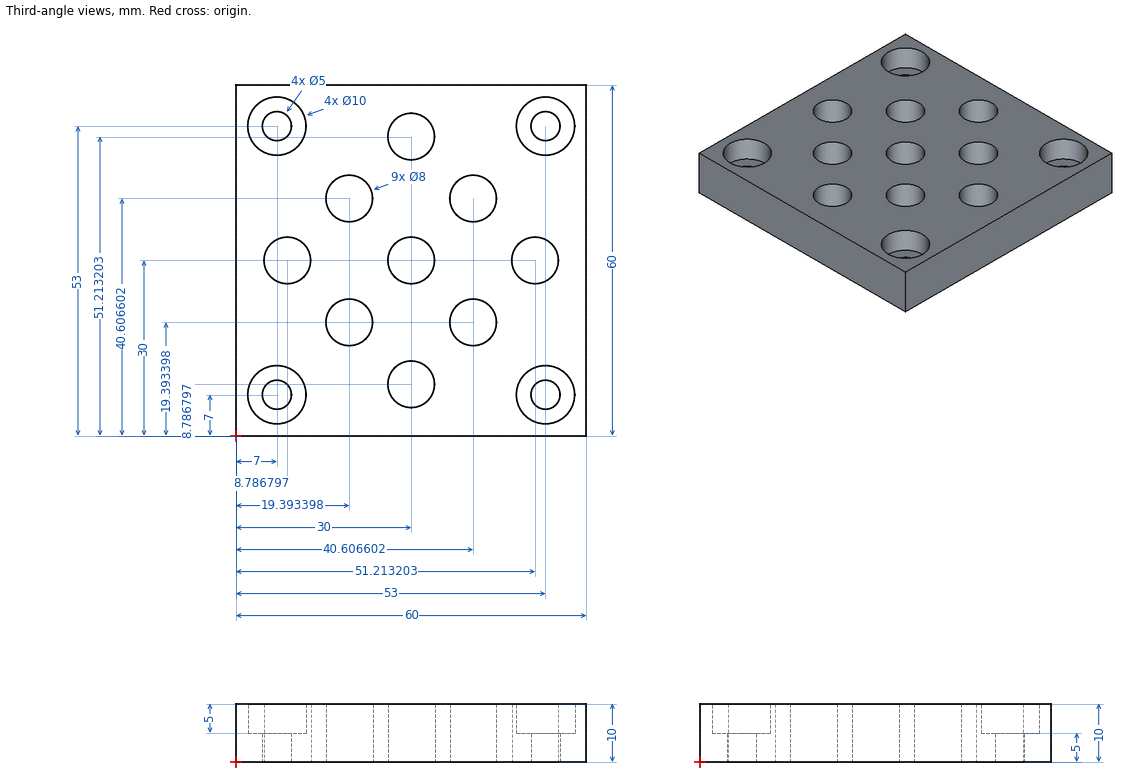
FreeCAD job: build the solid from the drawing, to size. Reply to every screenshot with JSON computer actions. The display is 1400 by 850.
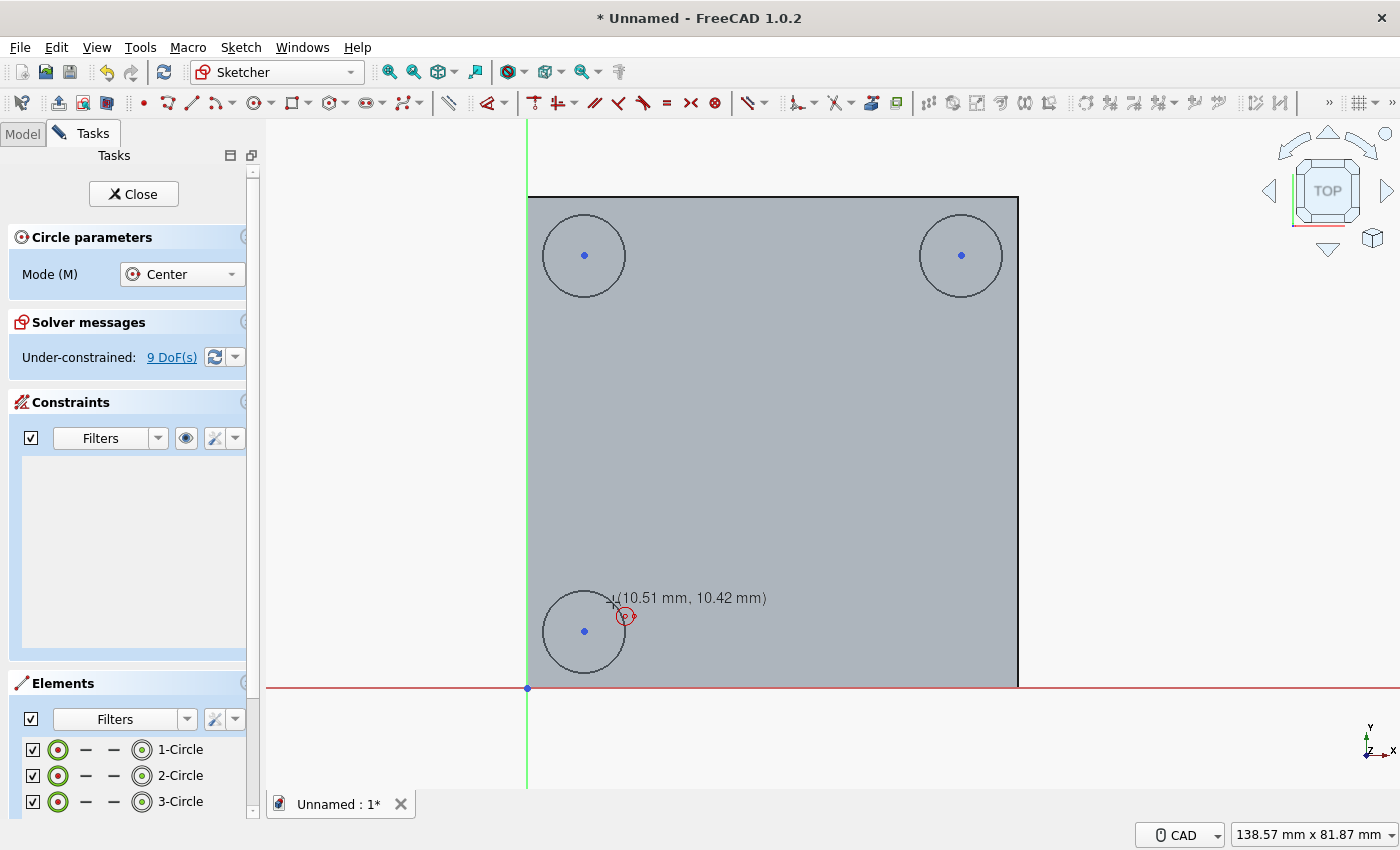
{"action": "left_click", "coordinate": [961, 631]}
{"action": "left_click", "coordinate": [990, 602]}
{"action": "key", "text": "Escape"}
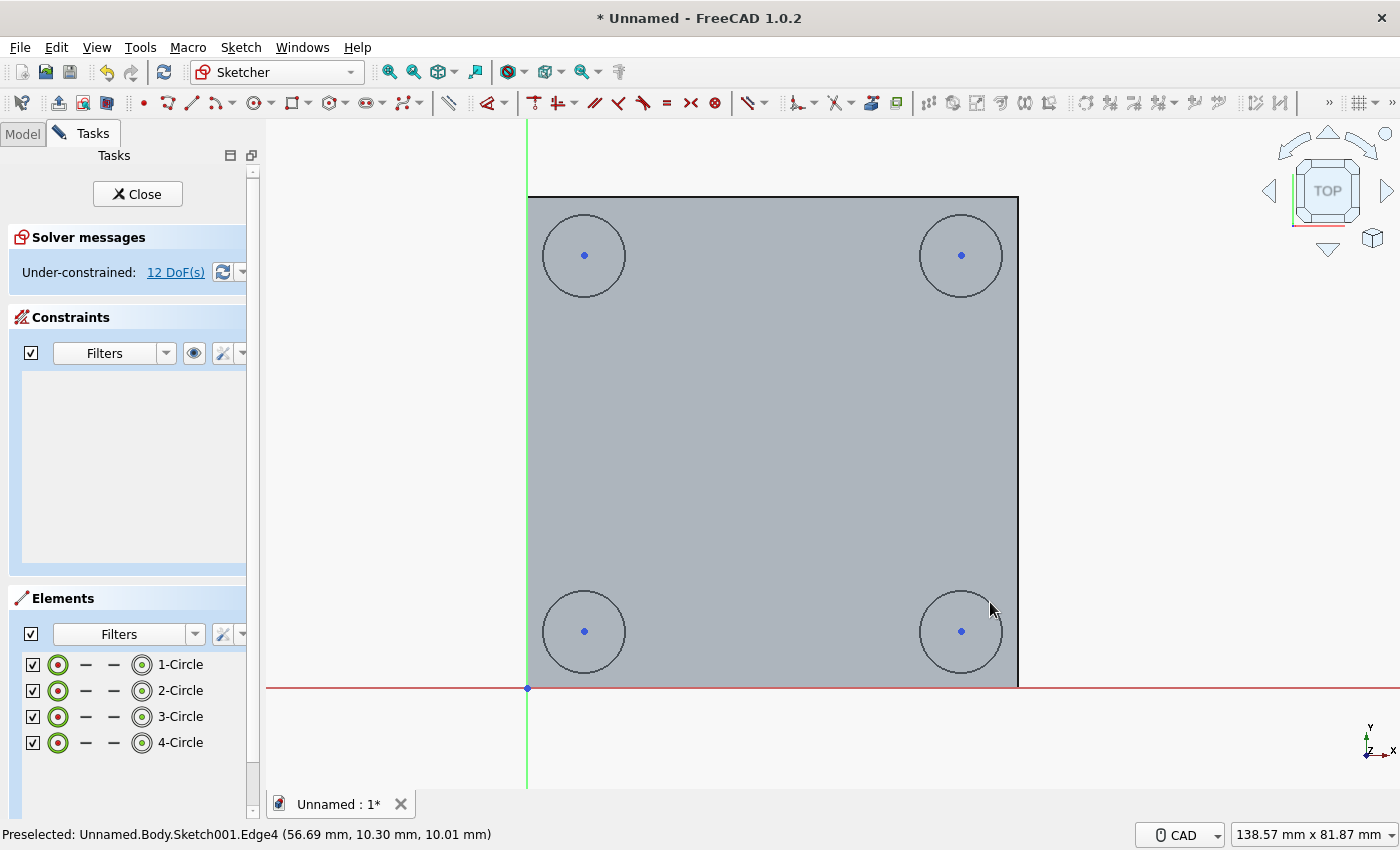
{"action": "left_click", "coordinate": [613, 227]}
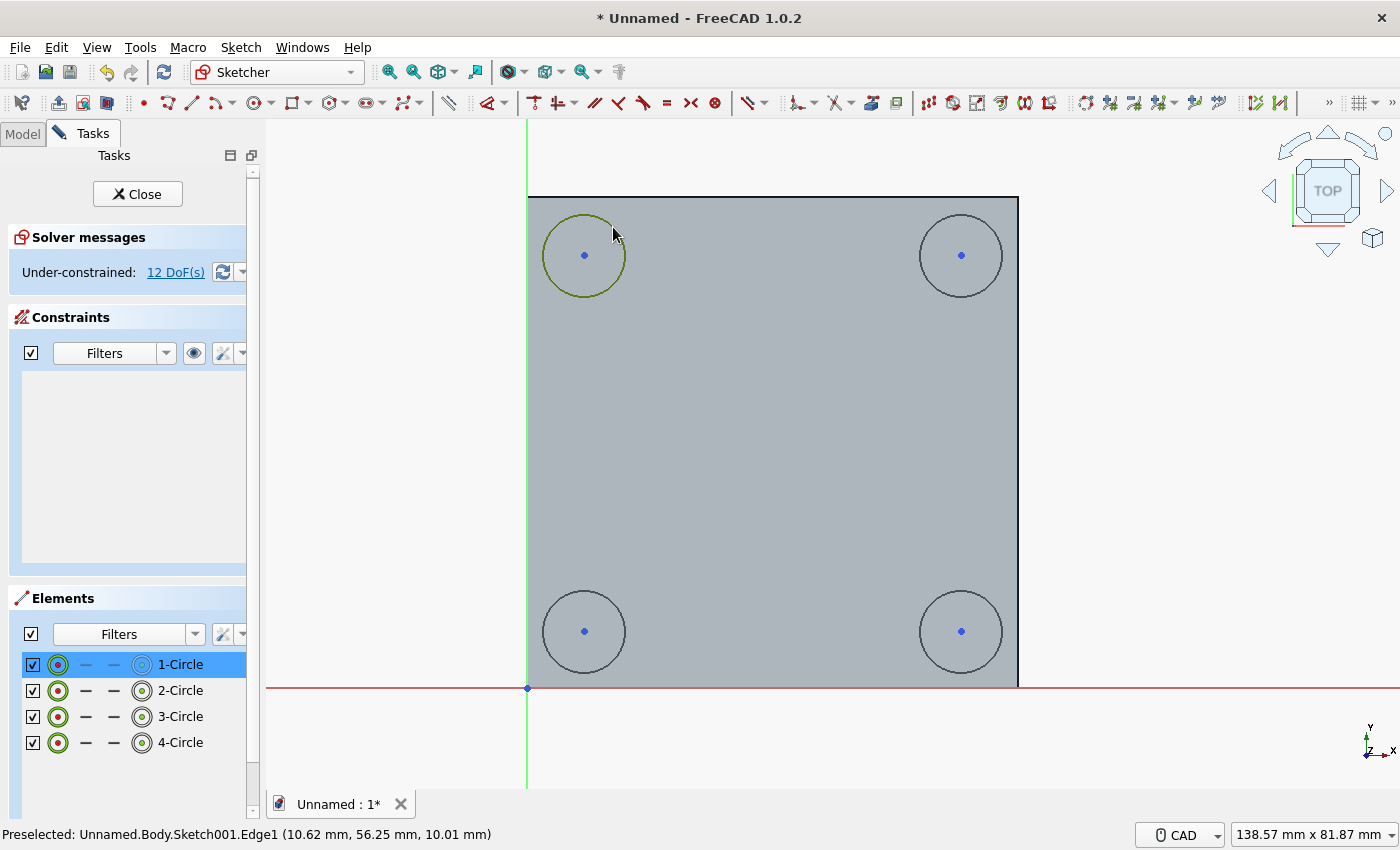
{"action": "left_click", "coordinate": [990, 227]}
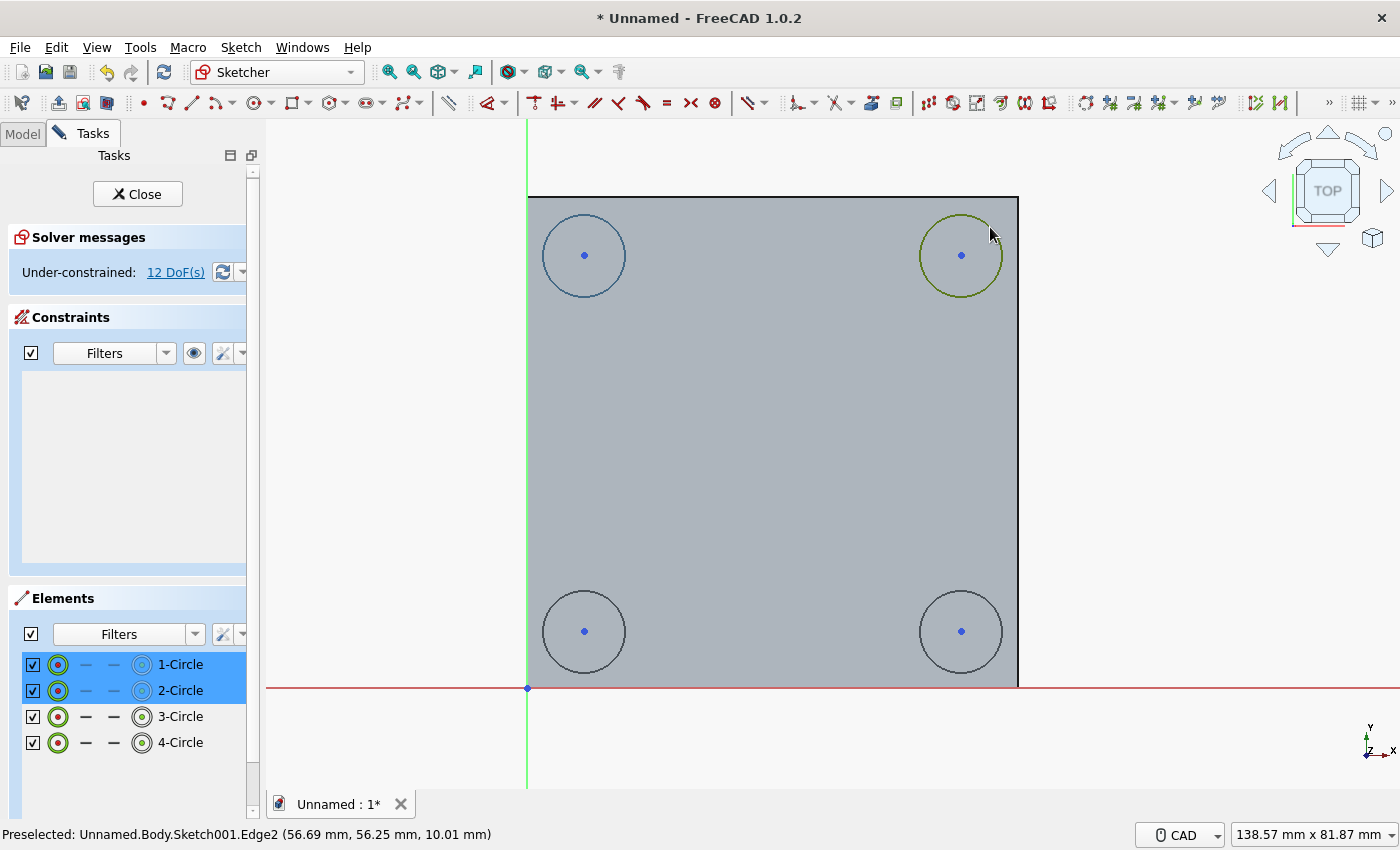
{"action": "left_click", "coordinate": [613, 603]}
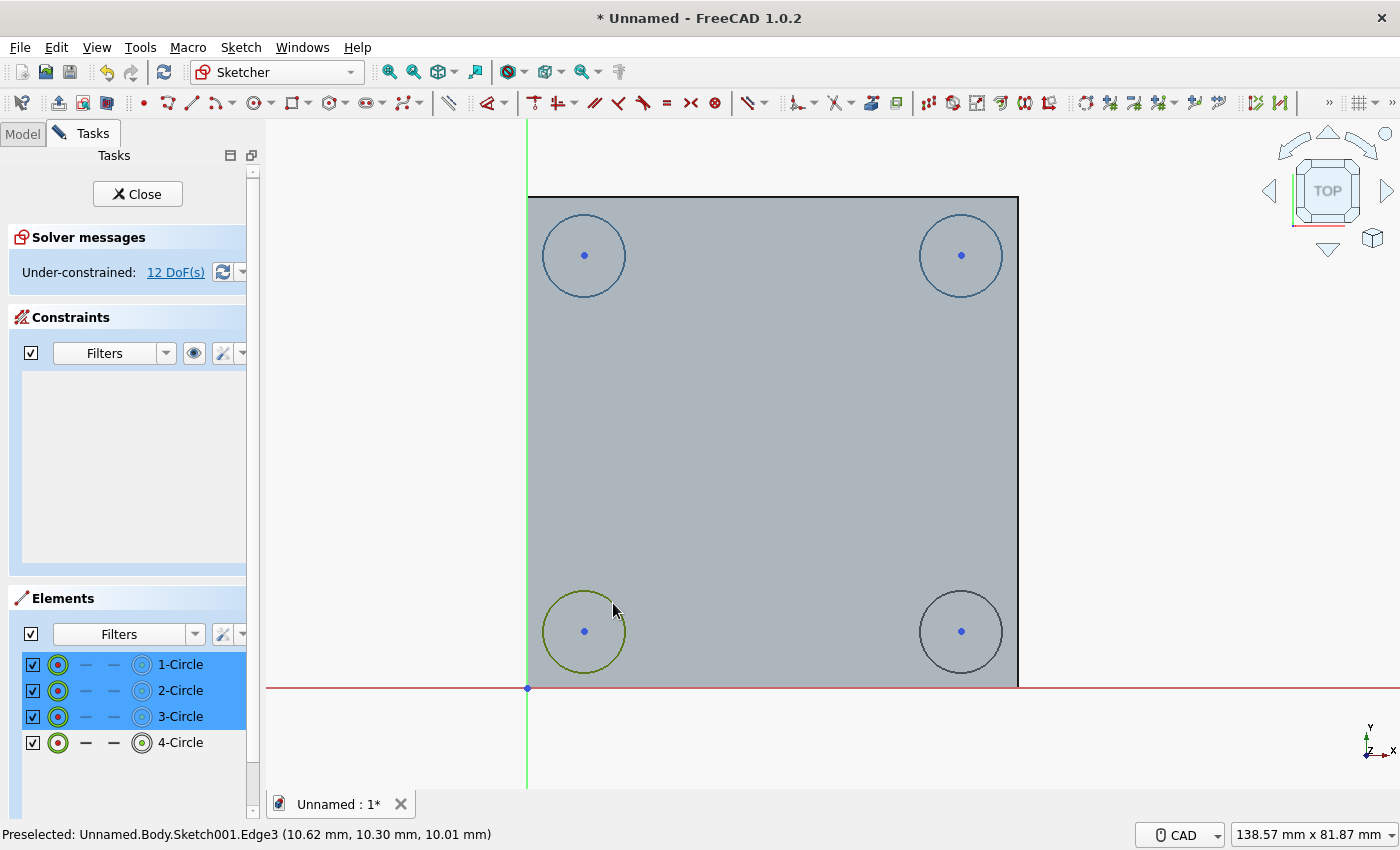
{"action": "left_click", "coordinate": [990, 603]}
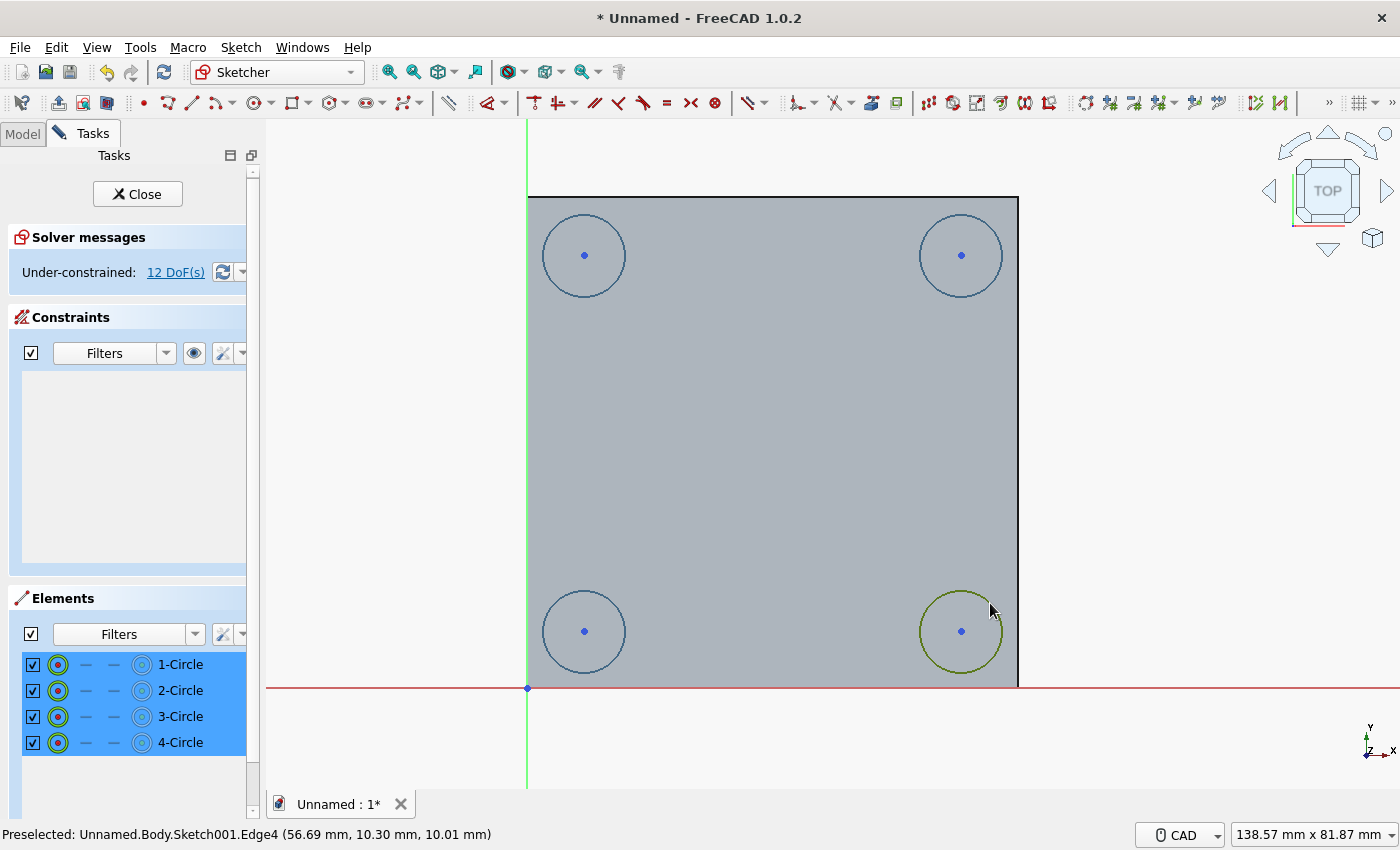
{"action": "key", "text": "e"}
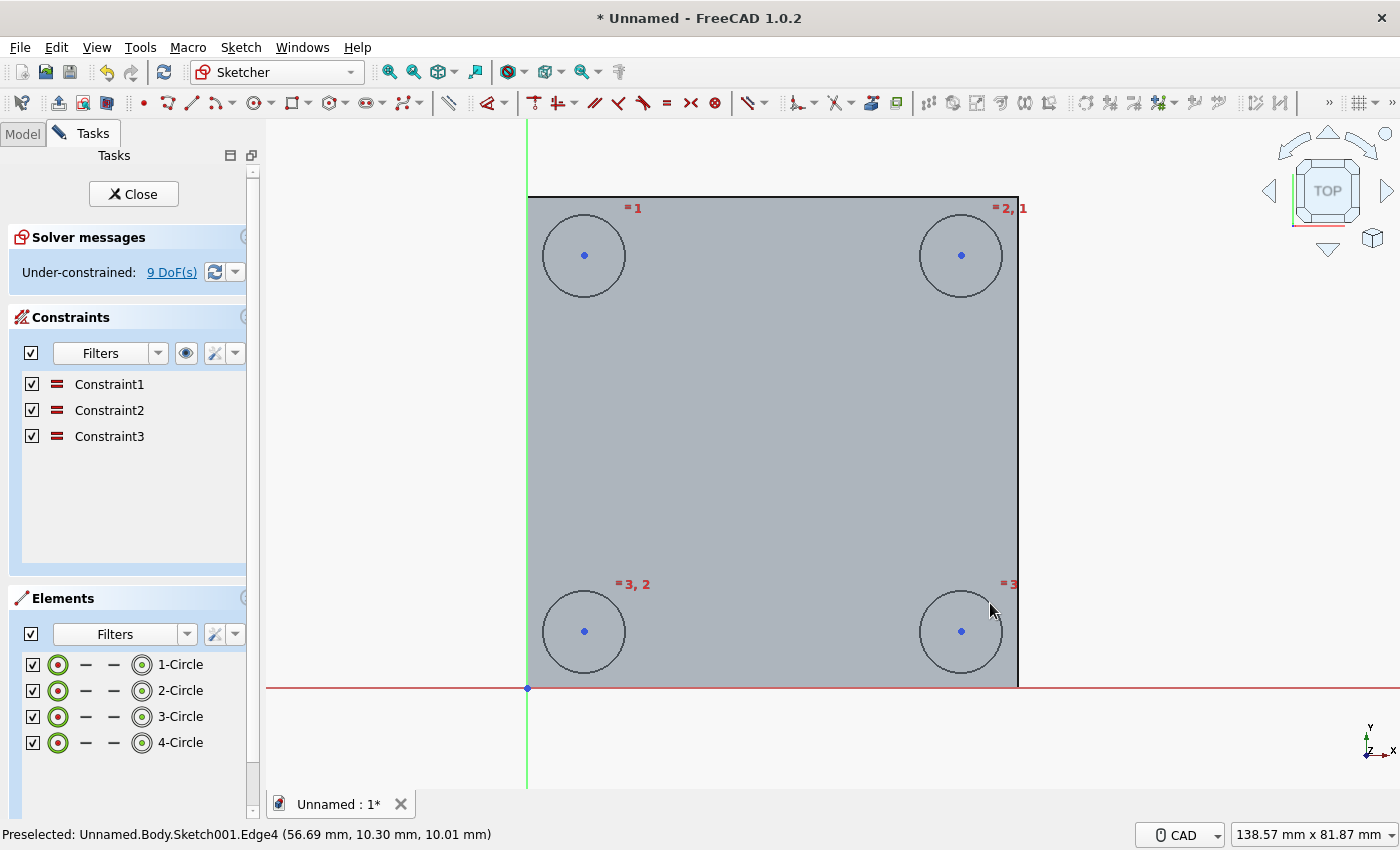
{"action": "left_click", "coordinate": [584, 256]}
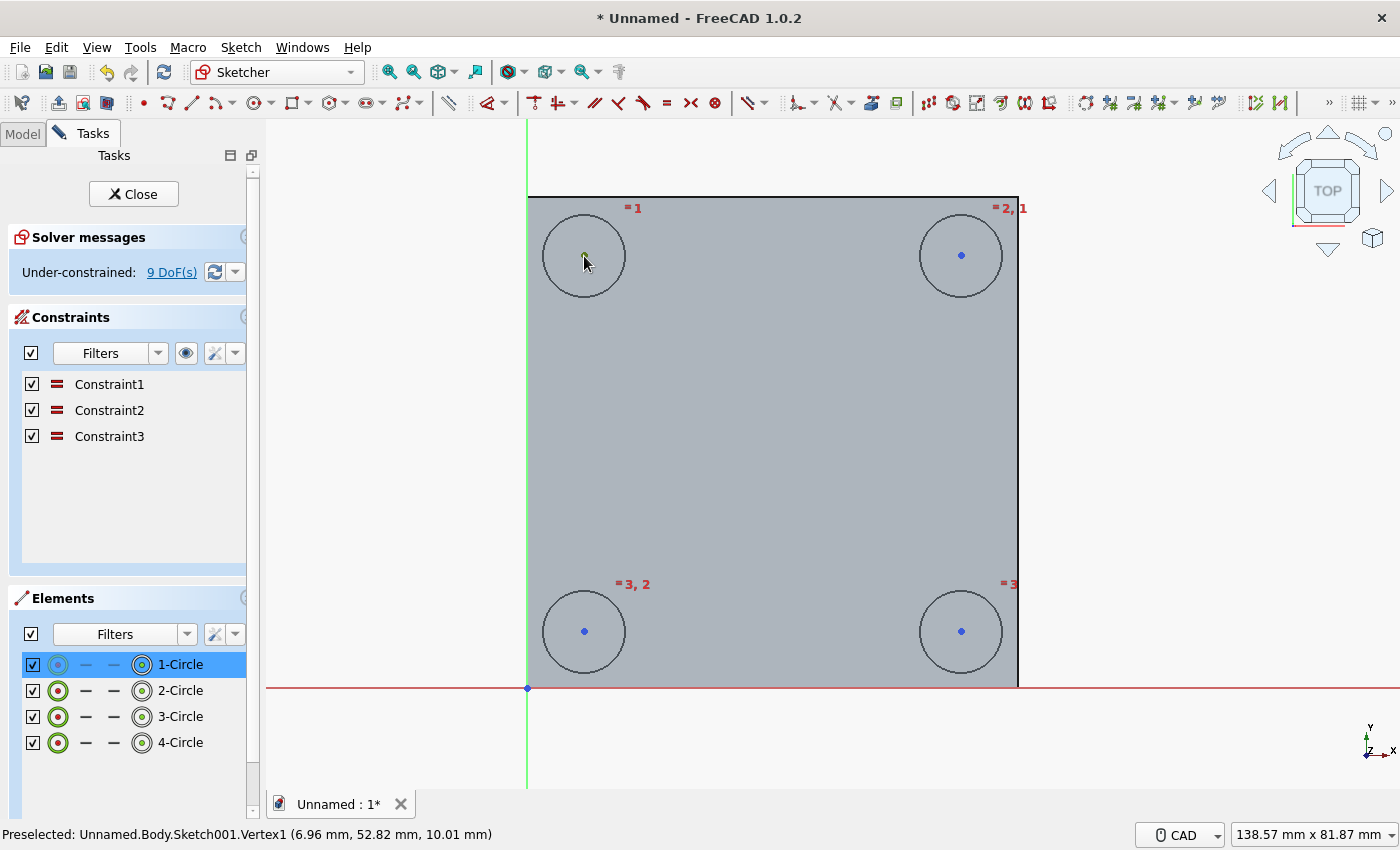
{"action": "left_click", "coordinate": [961, 256]}